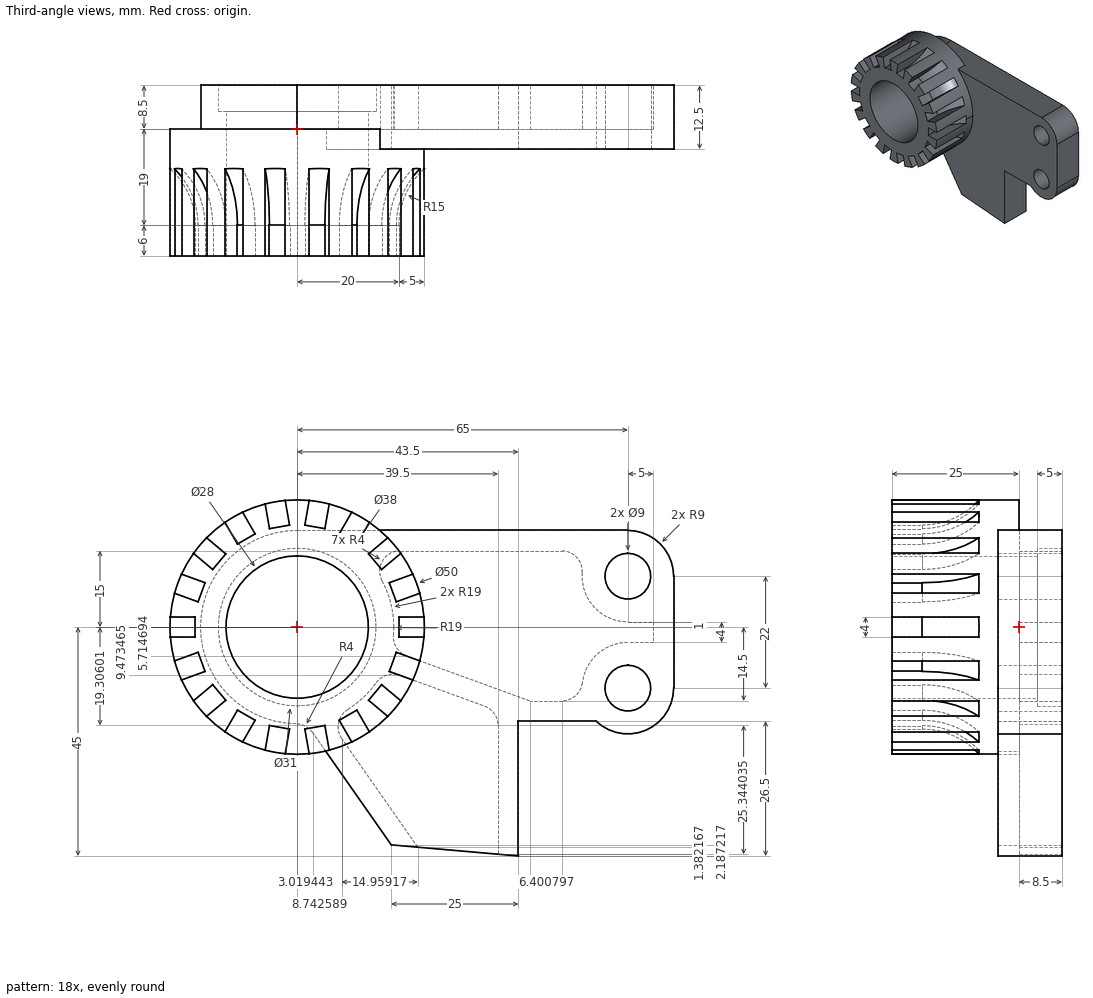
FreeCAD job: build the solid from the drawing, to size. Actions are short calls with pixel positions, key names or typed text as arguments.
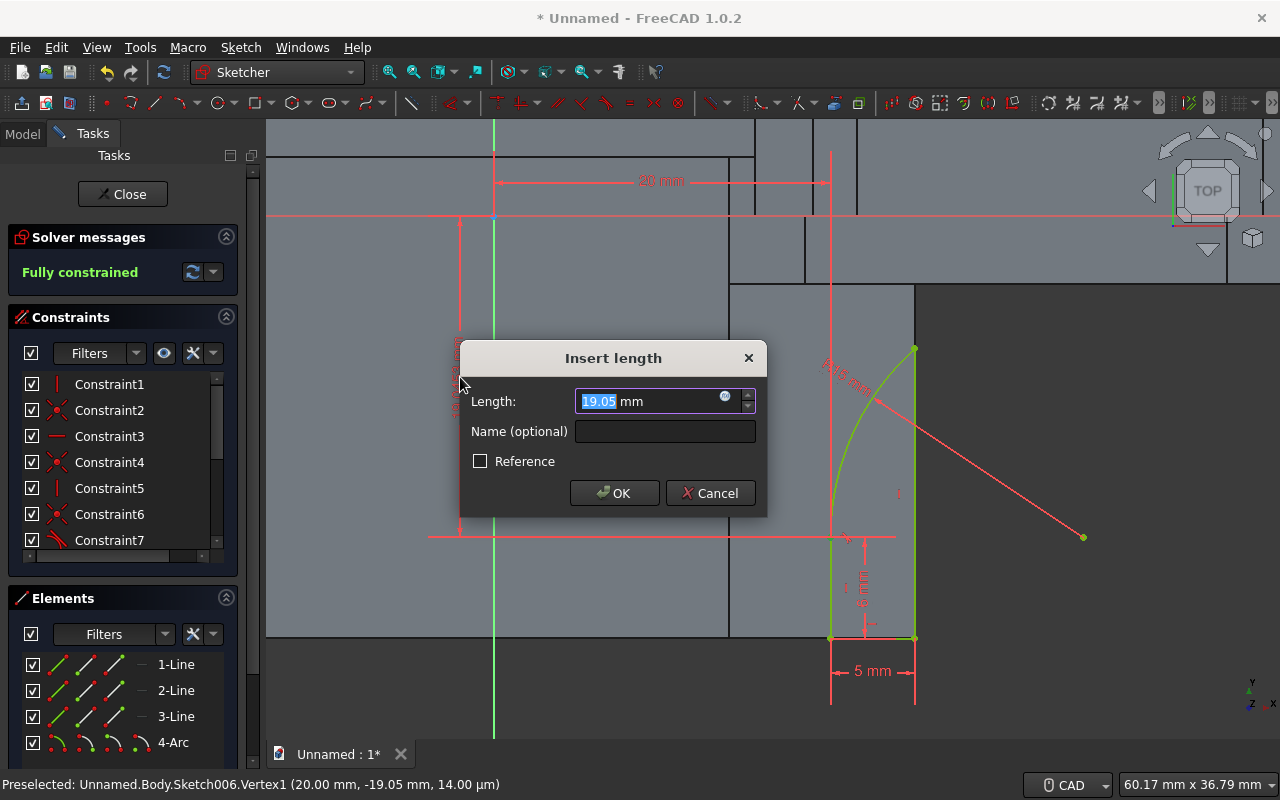
text(19)
key(Return)
key(Escape)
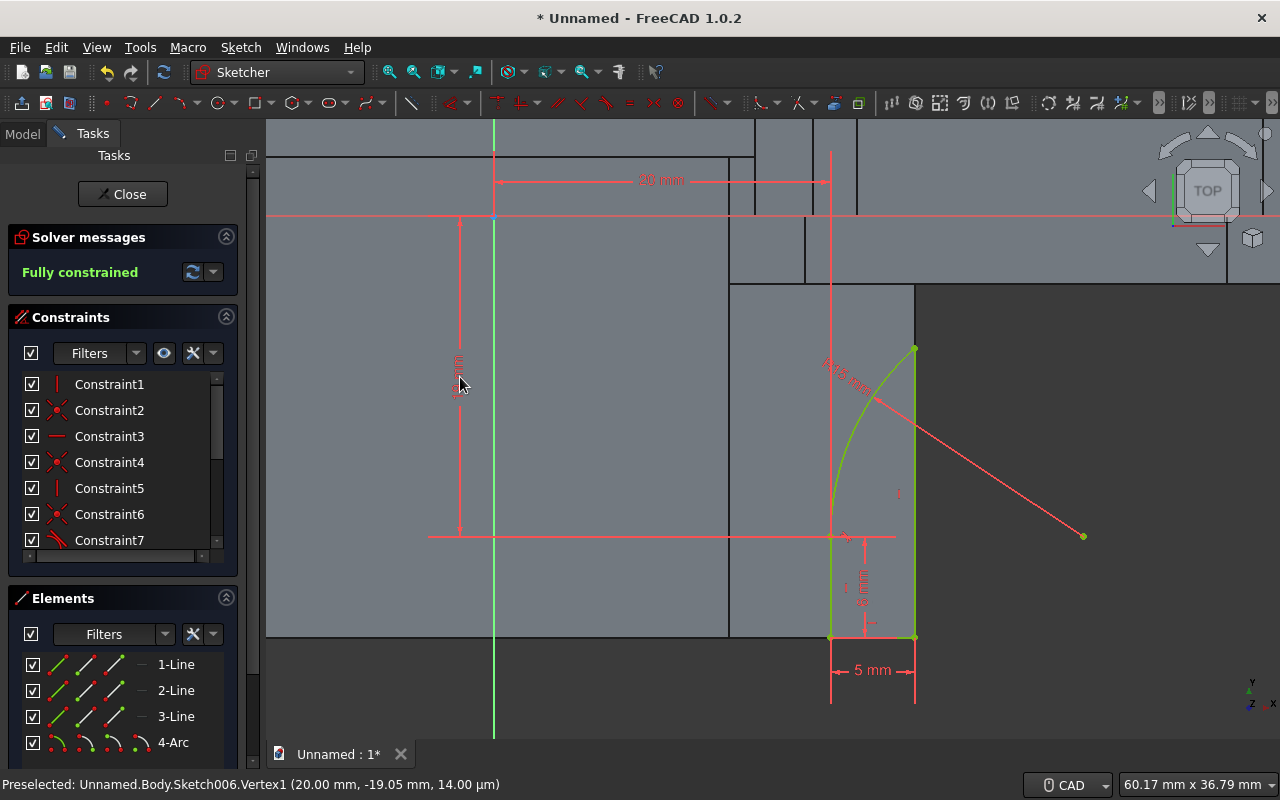
click(123, 194)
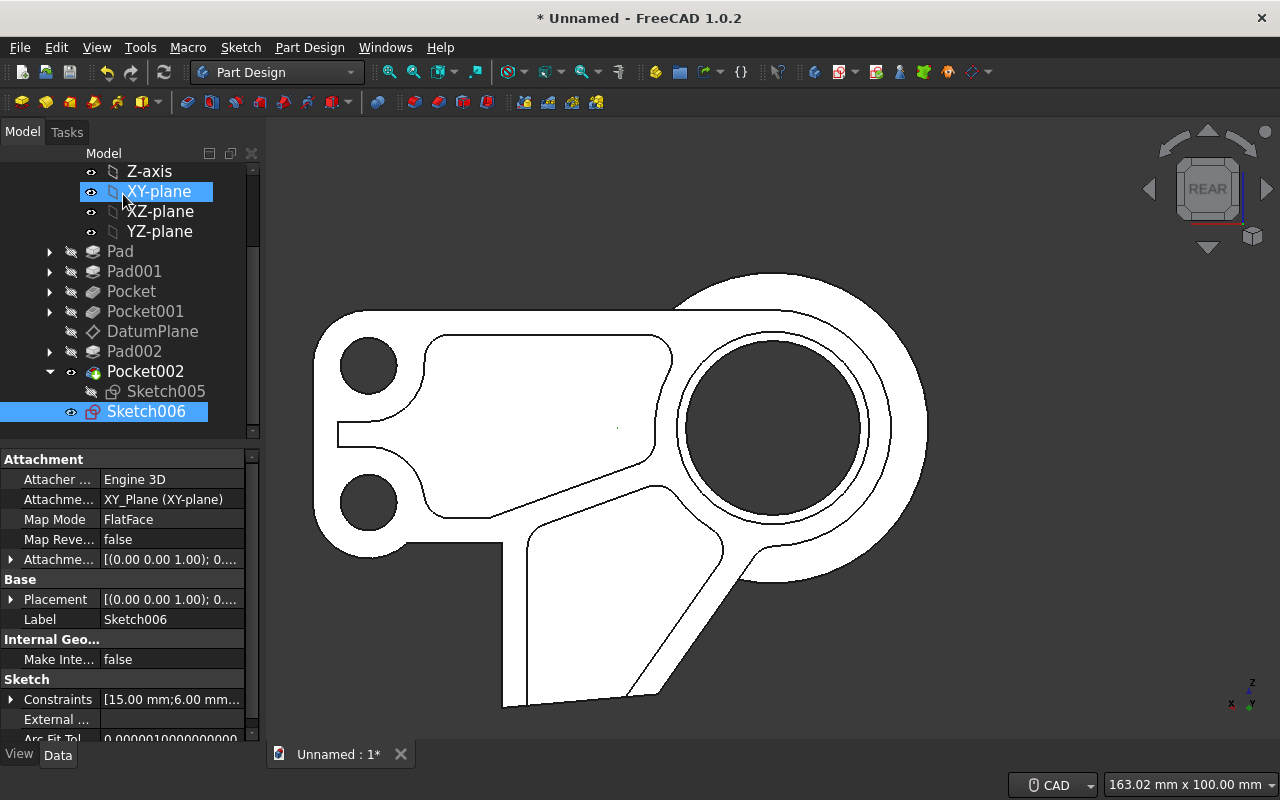
click(188, 102)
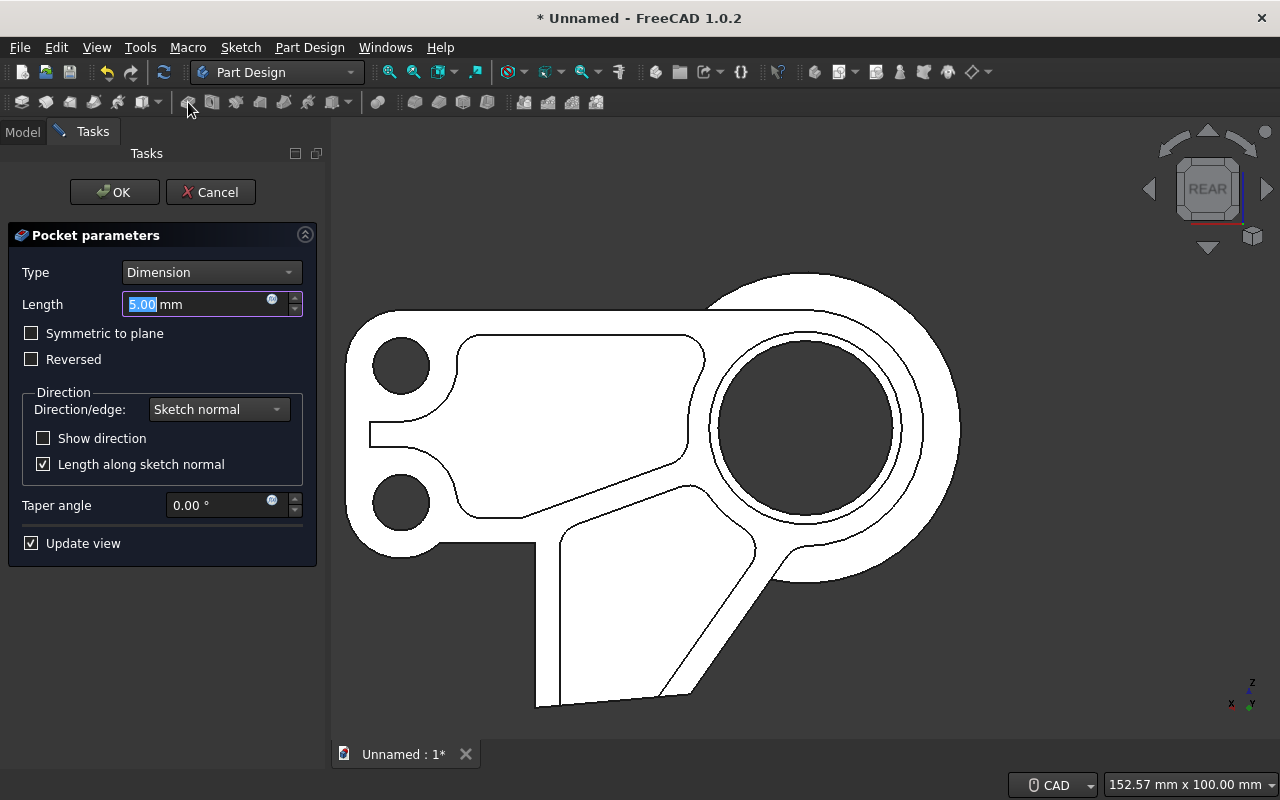
text(4)
key(Tab)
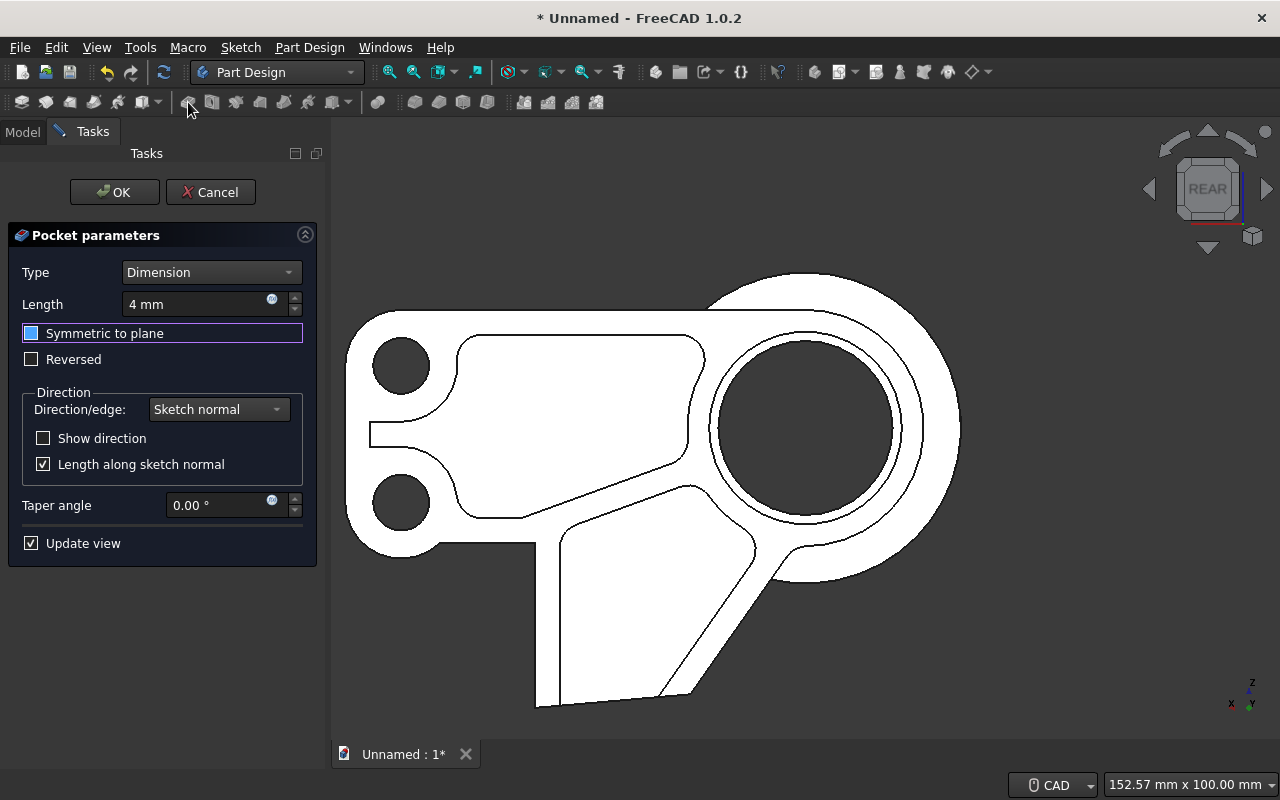
click(30, 333)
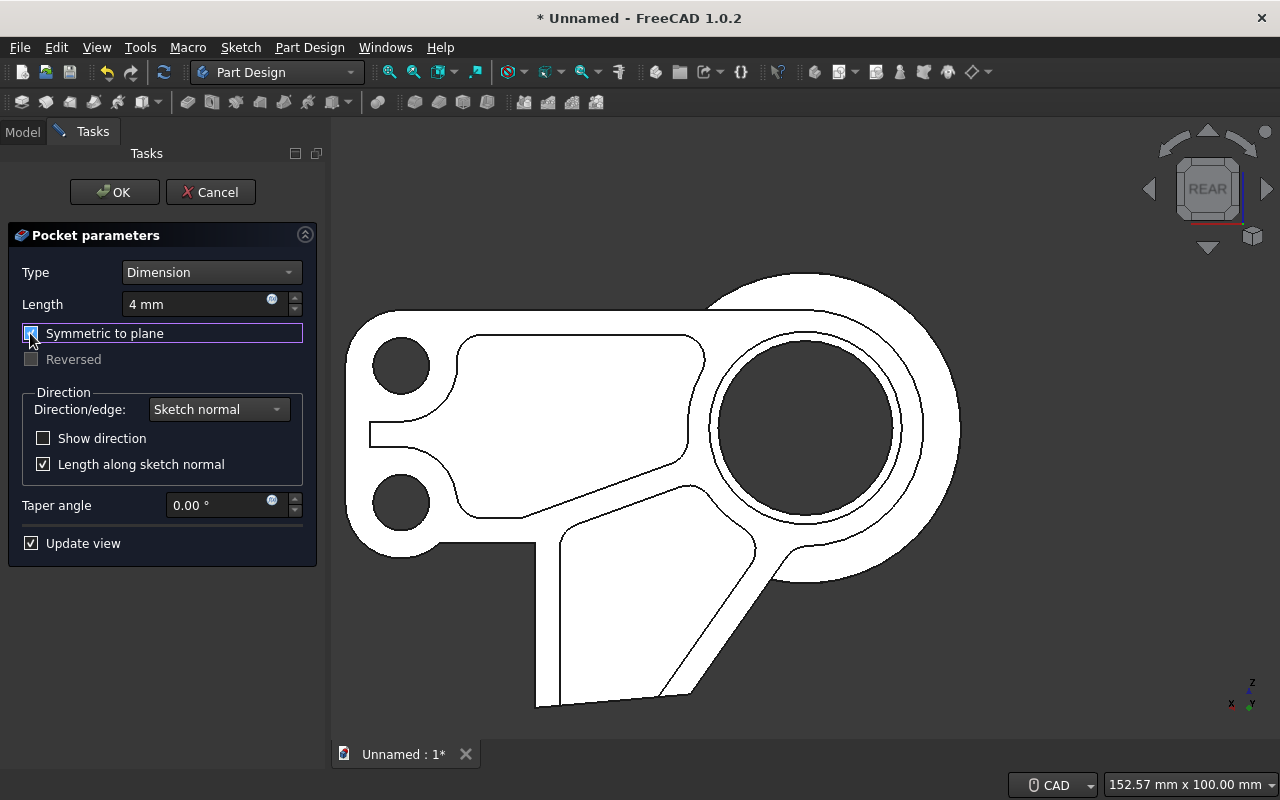
click(115, 192)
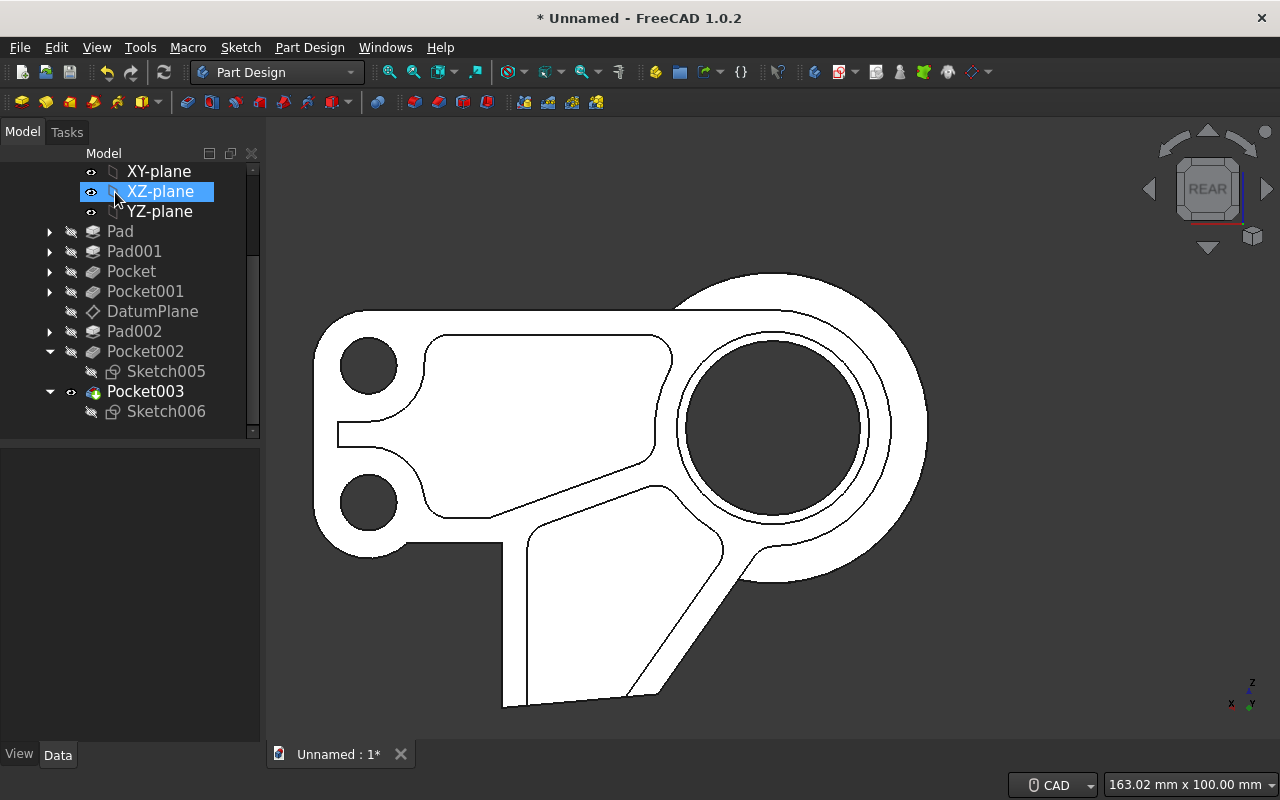
click(116, 392)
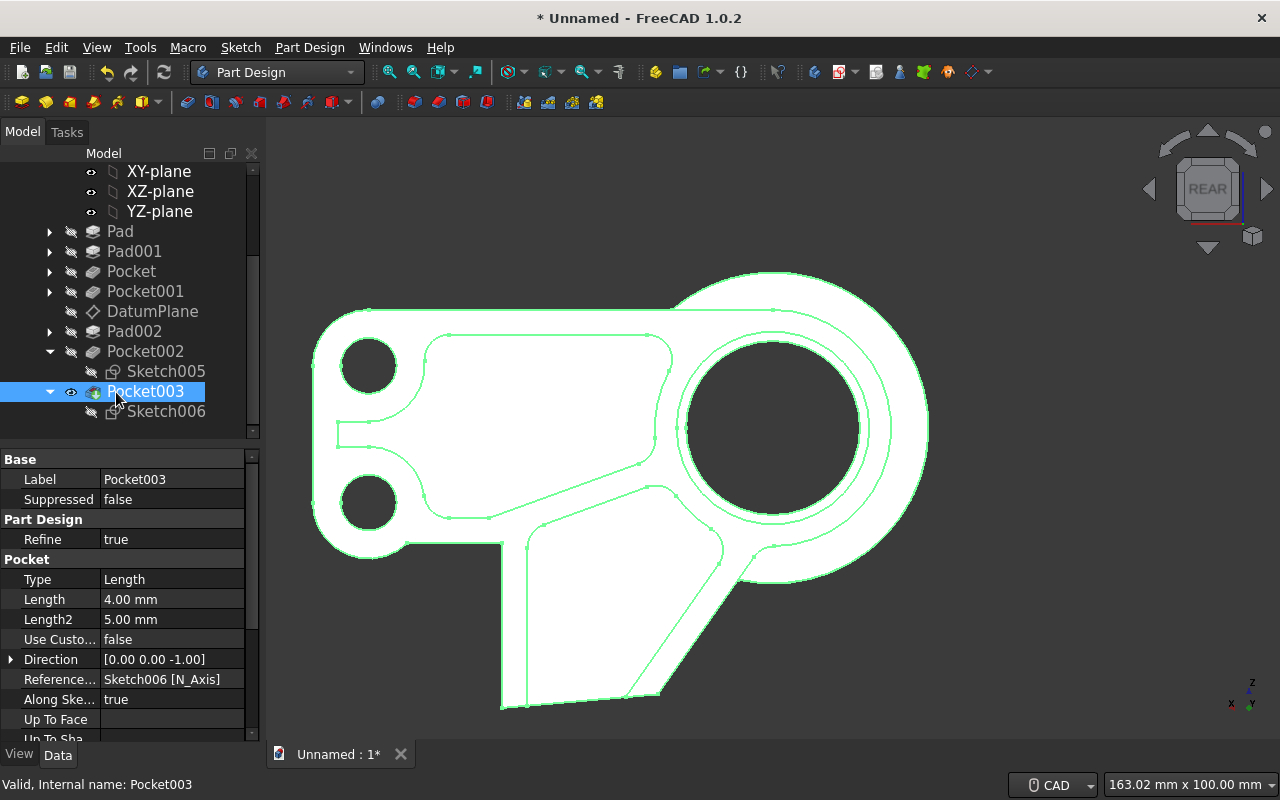
click(572, 102)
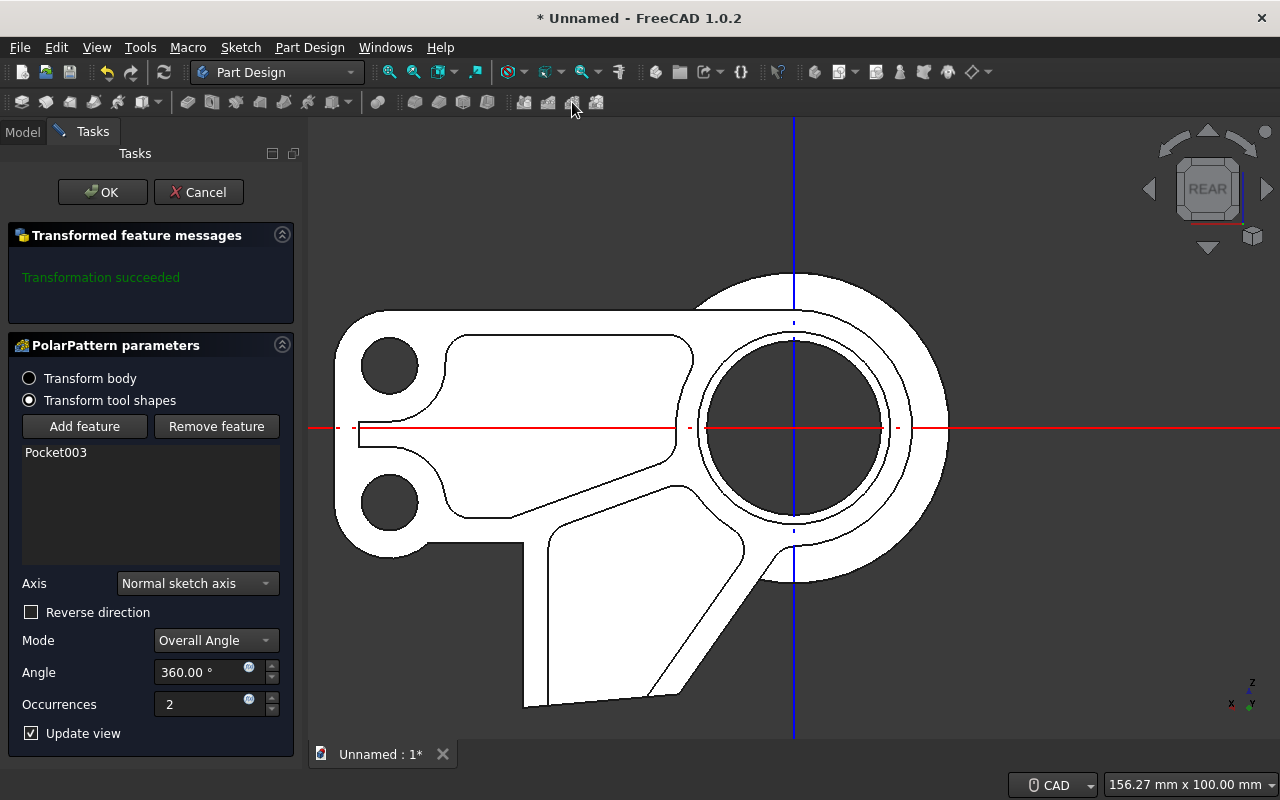
click(198, 584)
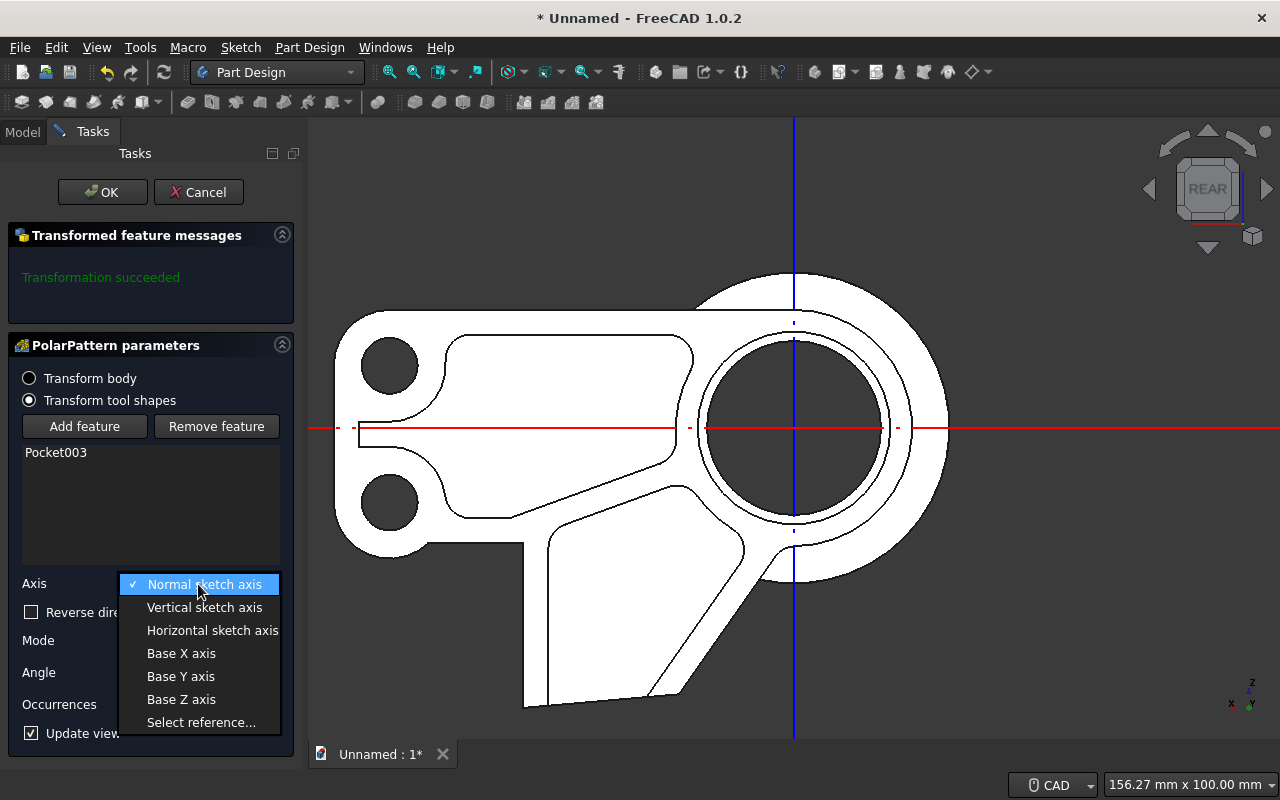
click(198, 676)